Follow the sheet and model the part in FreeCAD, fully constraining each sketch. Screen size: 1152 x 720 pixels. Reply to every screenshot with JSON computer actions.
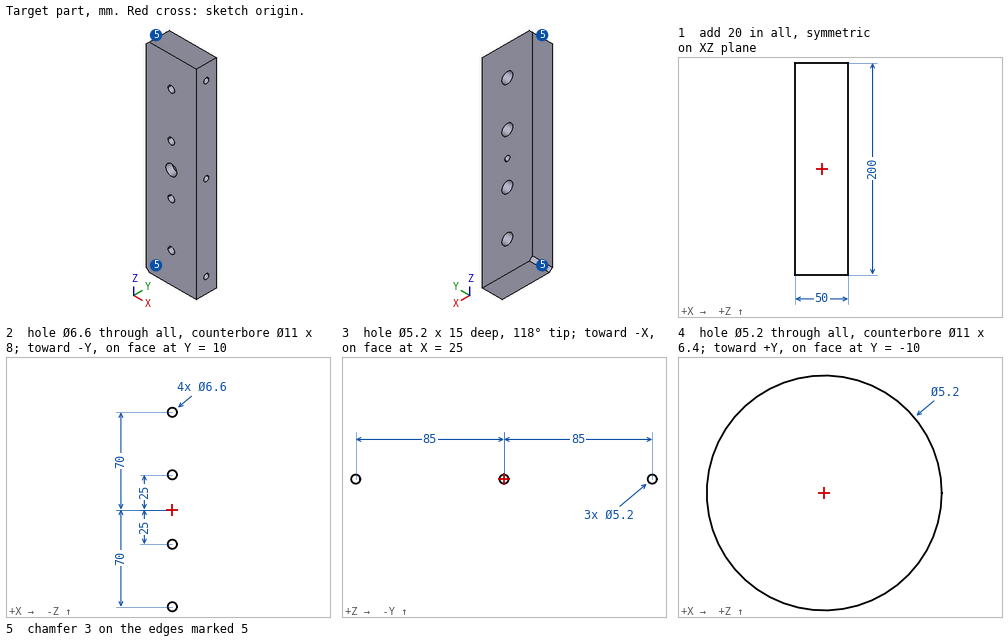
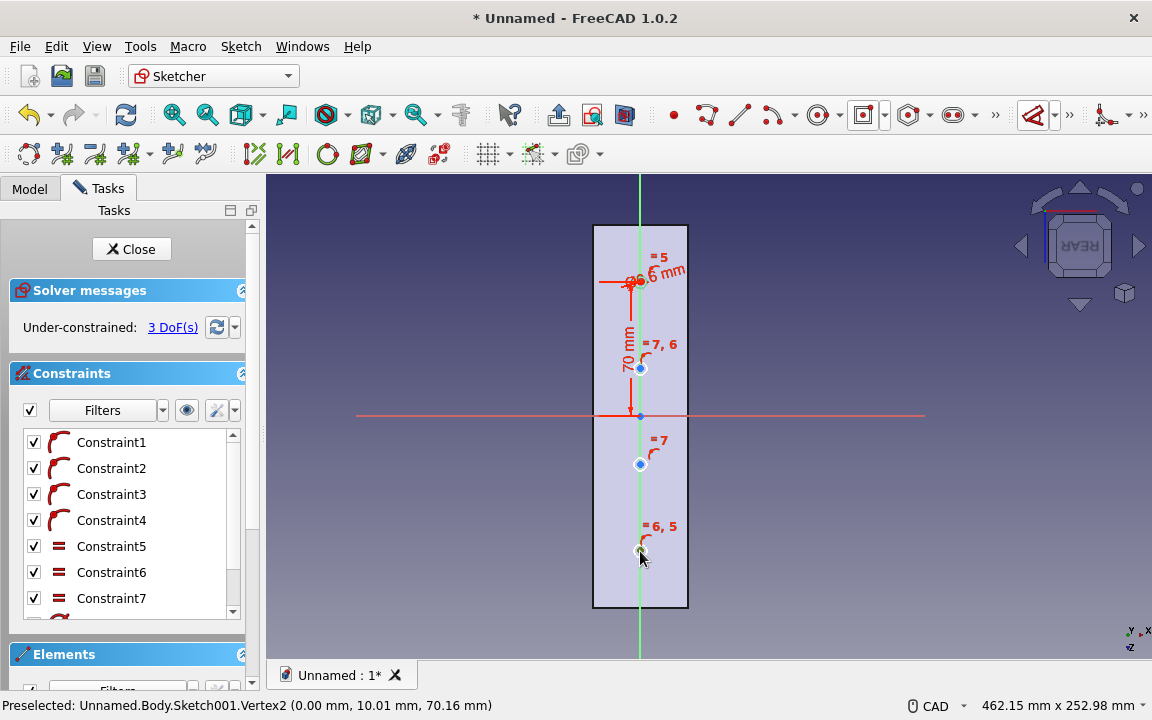
{"action": "key", "text": "i"}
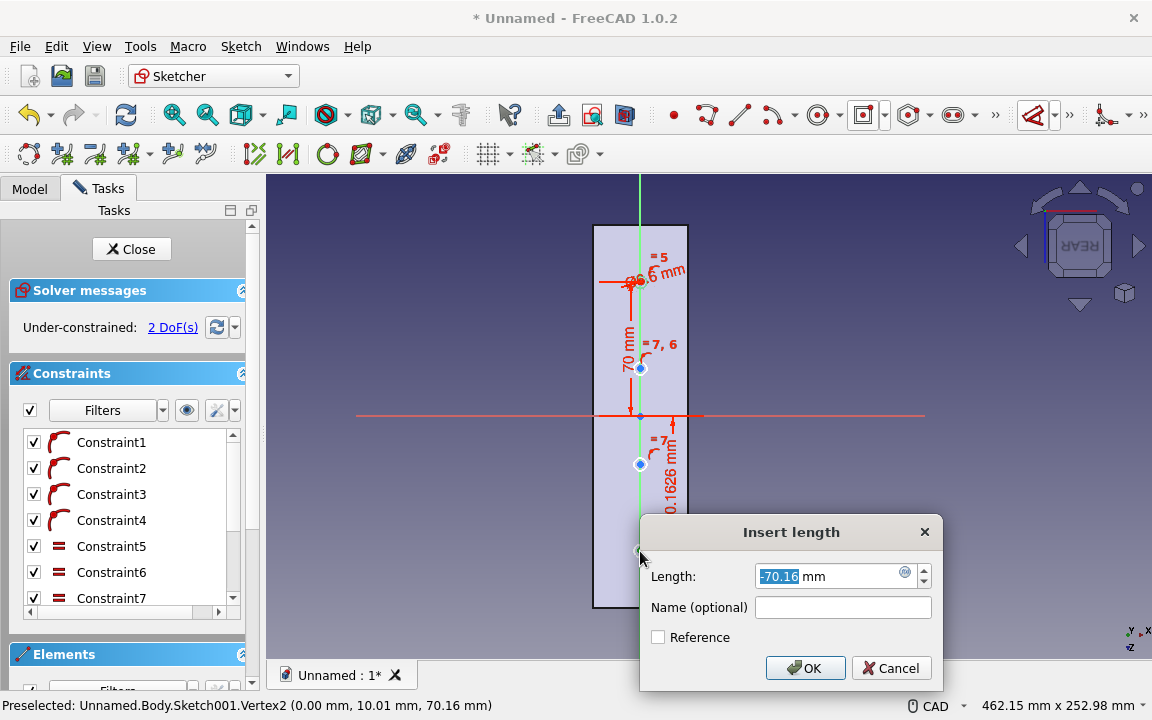
{"action": "type", "text": "-70"}
{"action": "key", "text": "Return"}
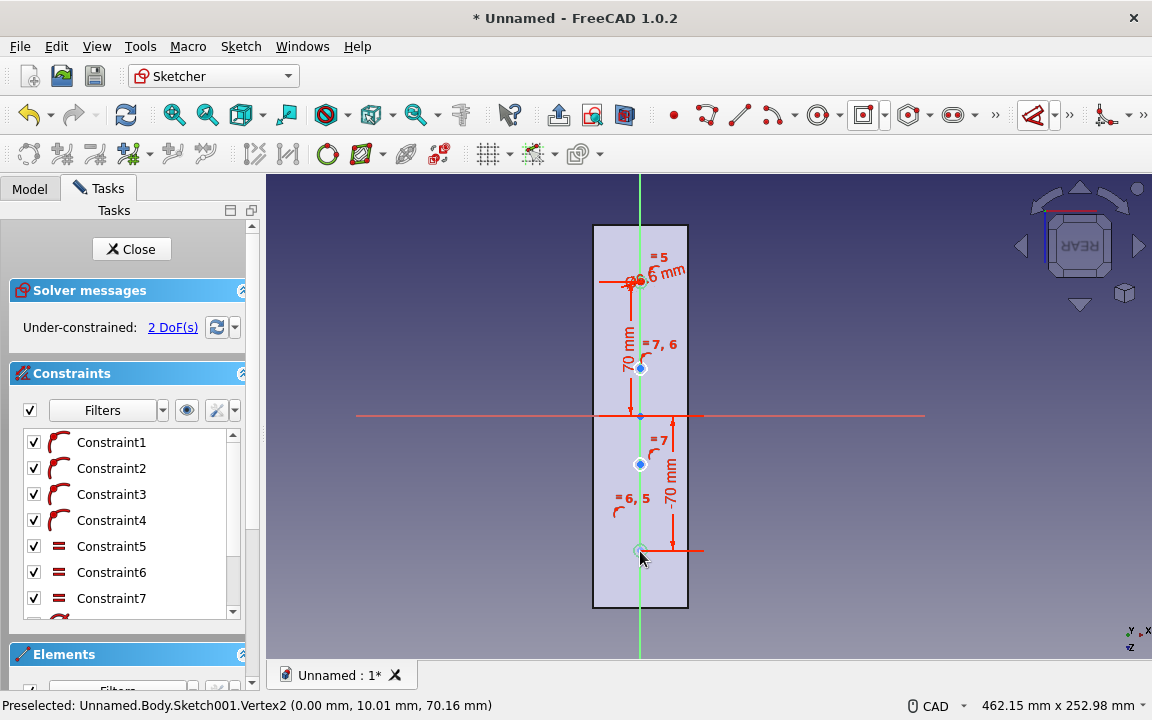
{"action": "left_click", "coordinate": [640, 369]}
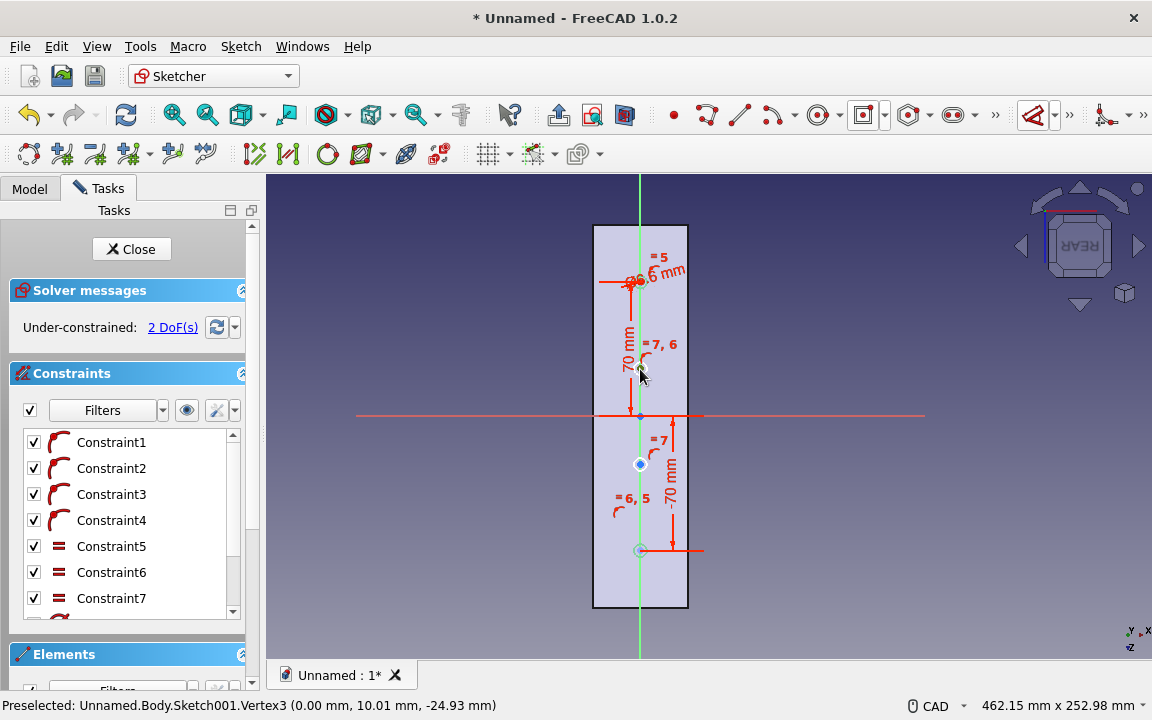
{"action": "left_click", "coordinate": [1054, 116]}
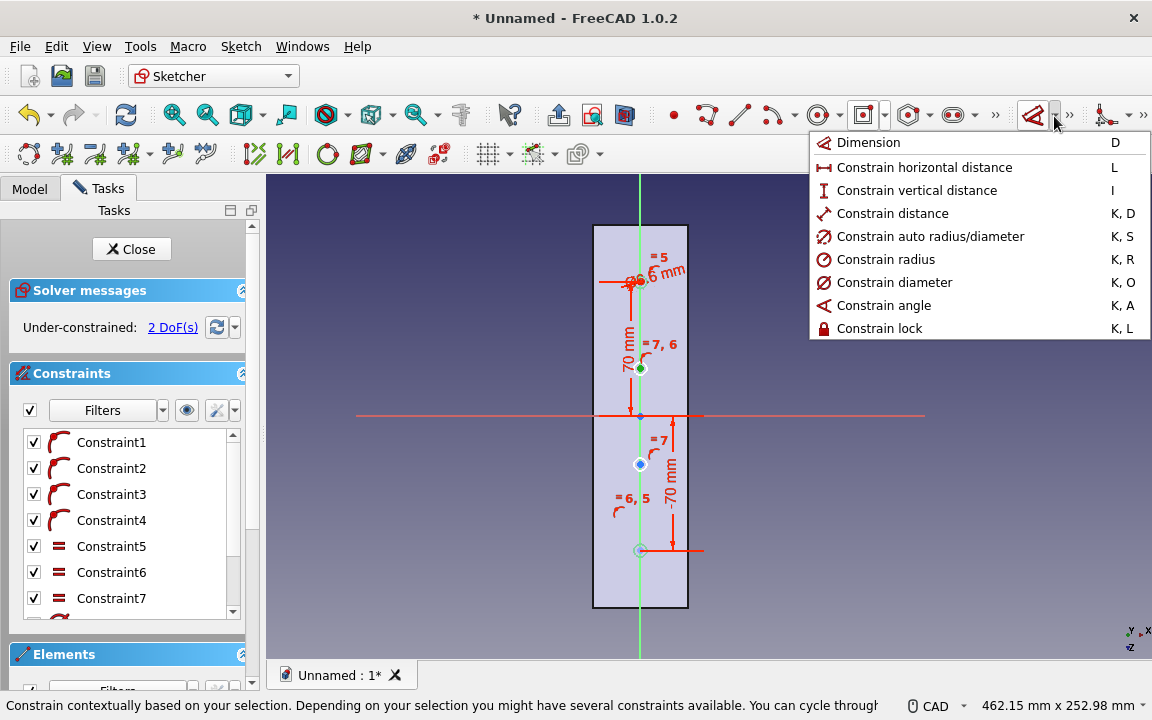
{"action": "left_click", "coordinate": [980, 190]}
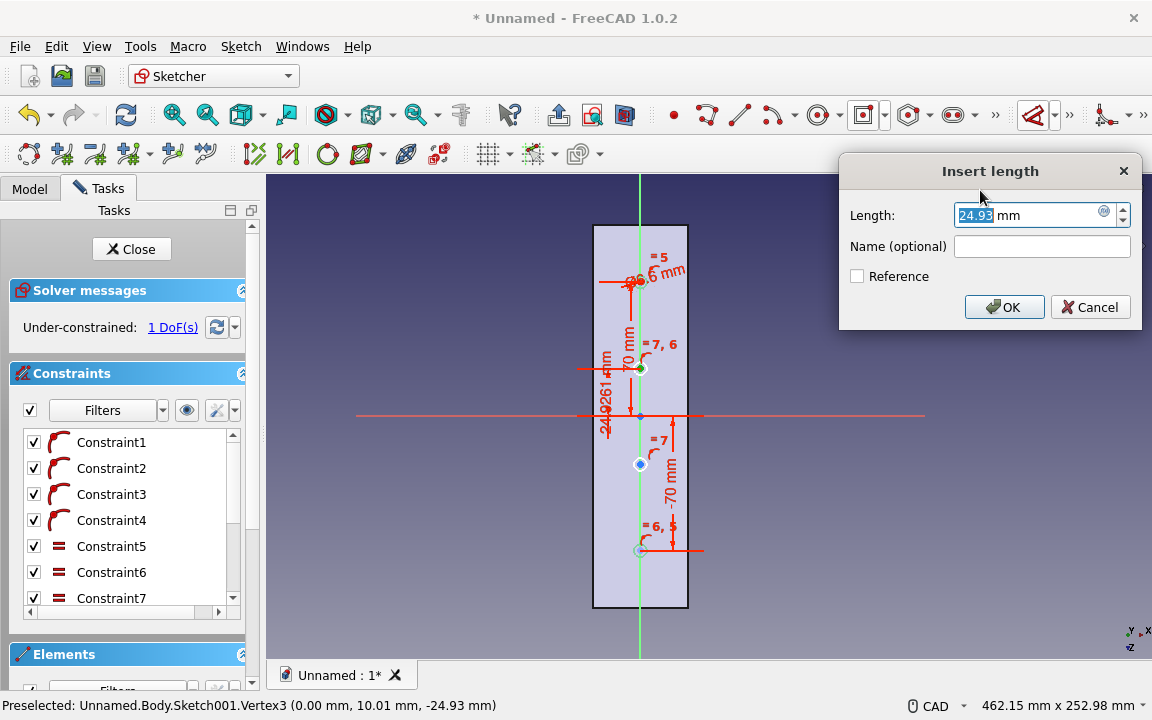
{"action": "type", "text": "25"}
{"action": "key", "text": "Return"}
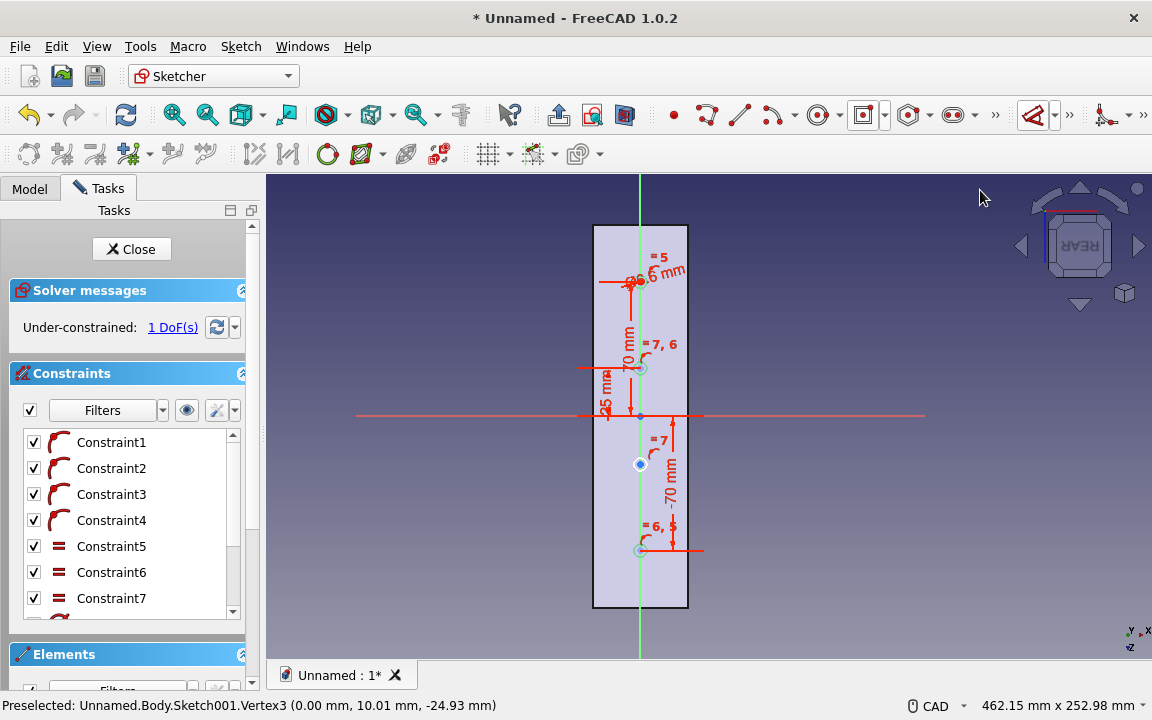
{"action": "left_click", "coordinate": [640, 465]}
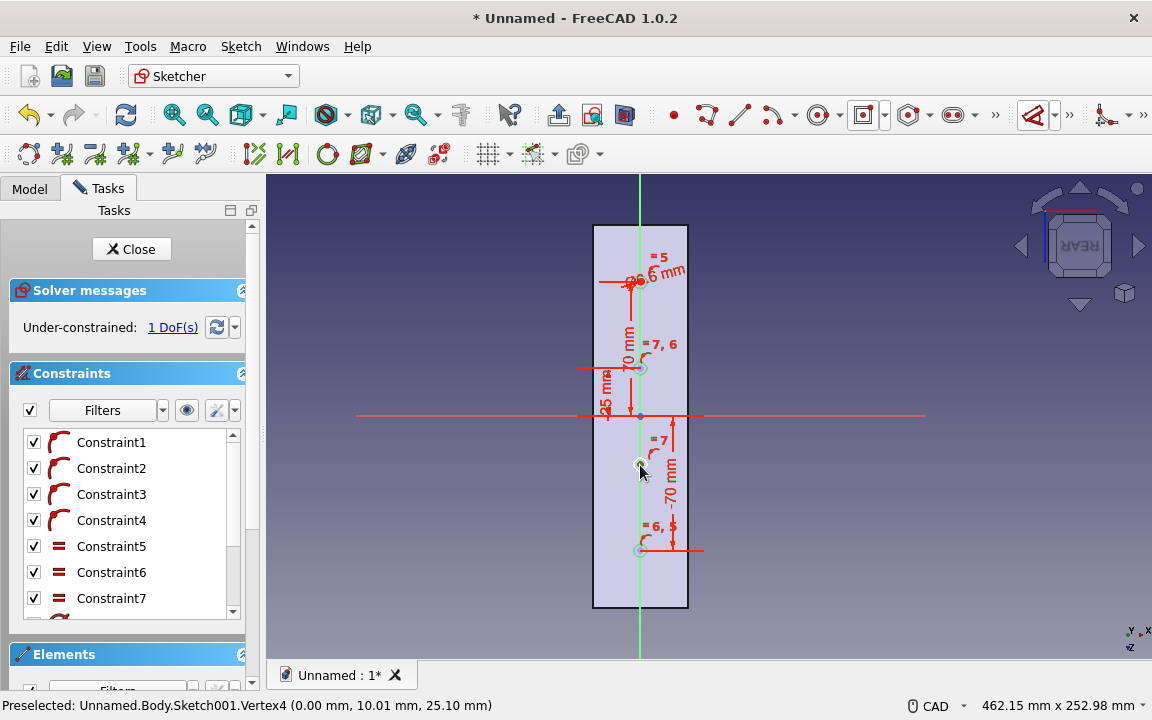
{"action": "left_click", "coordinate": [1054, 116]}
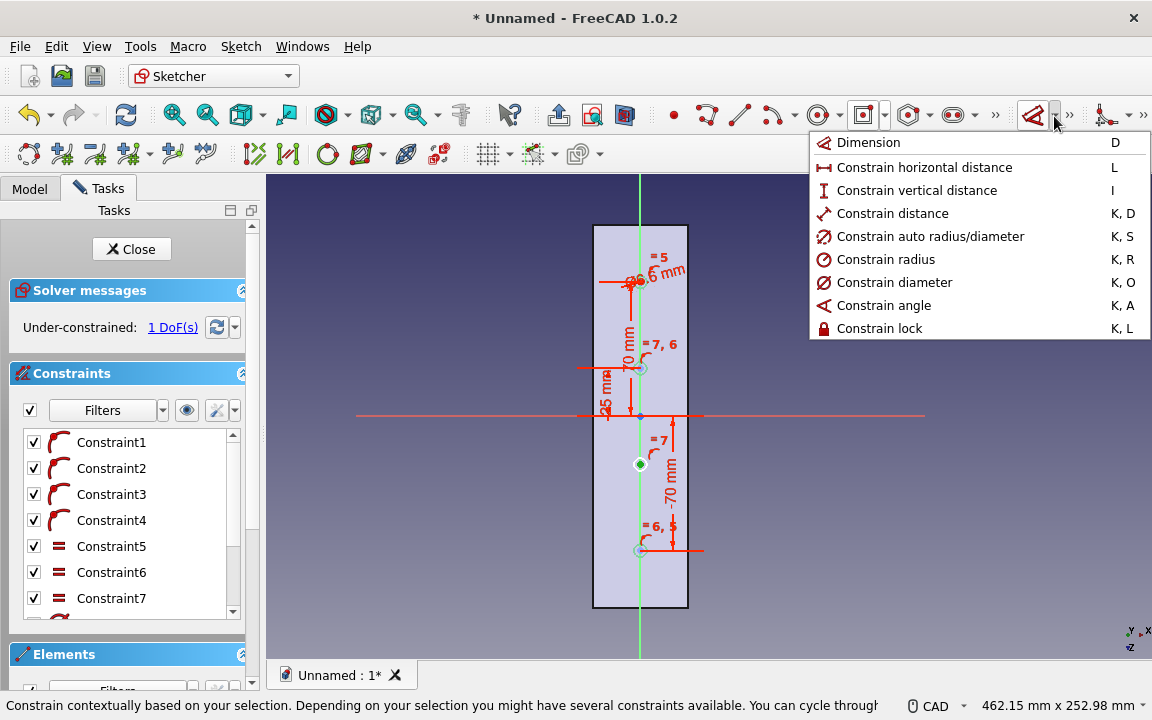
{"action": "left_click", "coordinate": [980, 190]}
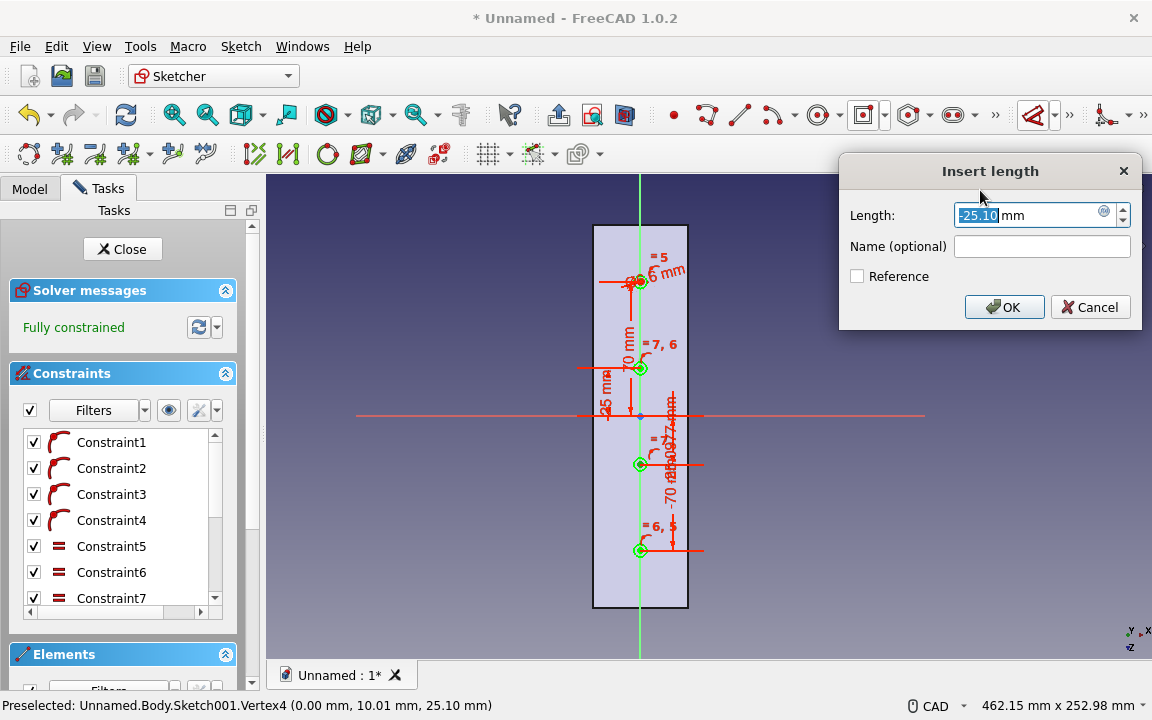
{"action": "type", "text": "-25"}
{"action": "key", "text": "Return"}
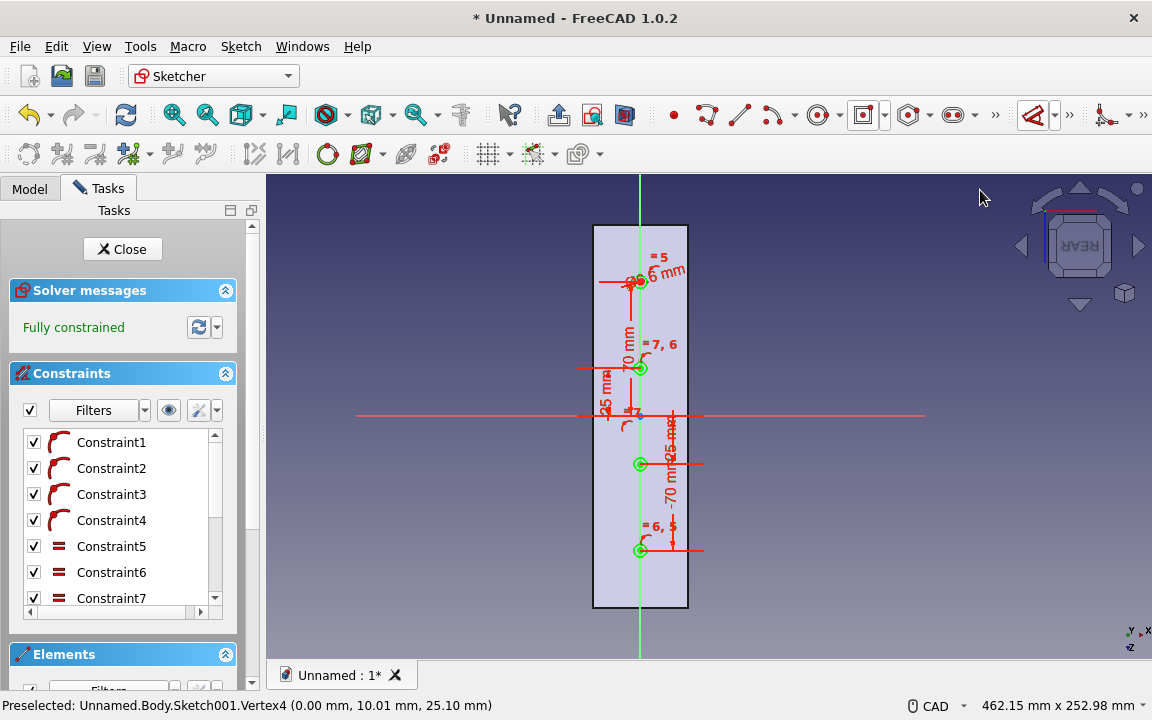
{"action": "left_click", "coordinate": [123, 249]}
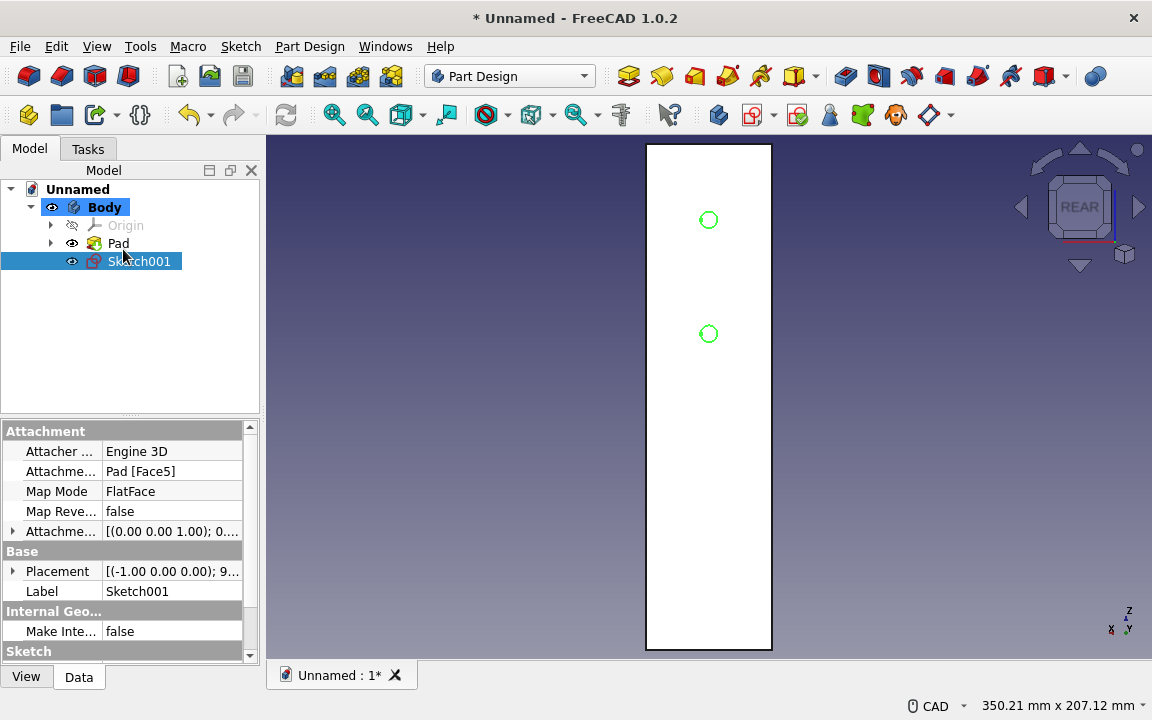
{"action": "left_click", "coordinate": [879, 76]}